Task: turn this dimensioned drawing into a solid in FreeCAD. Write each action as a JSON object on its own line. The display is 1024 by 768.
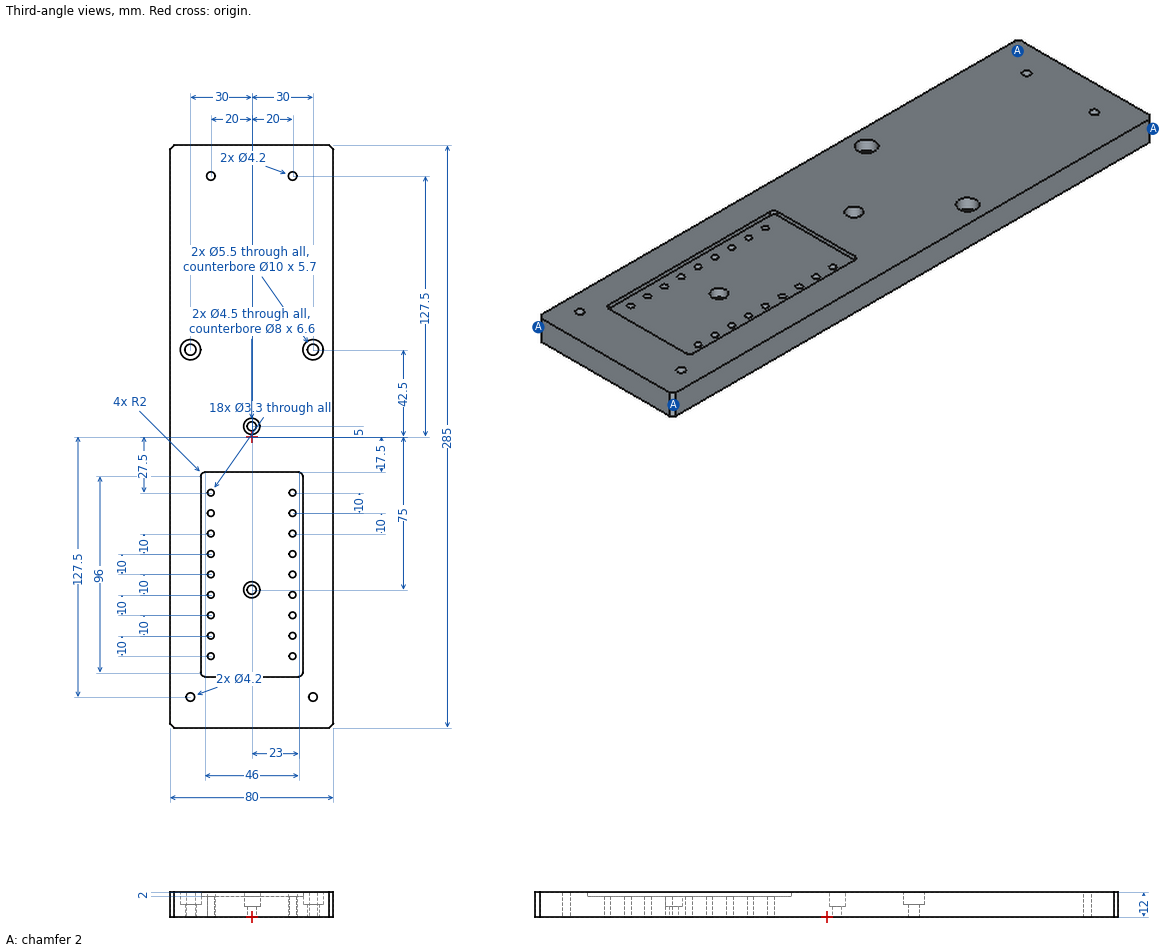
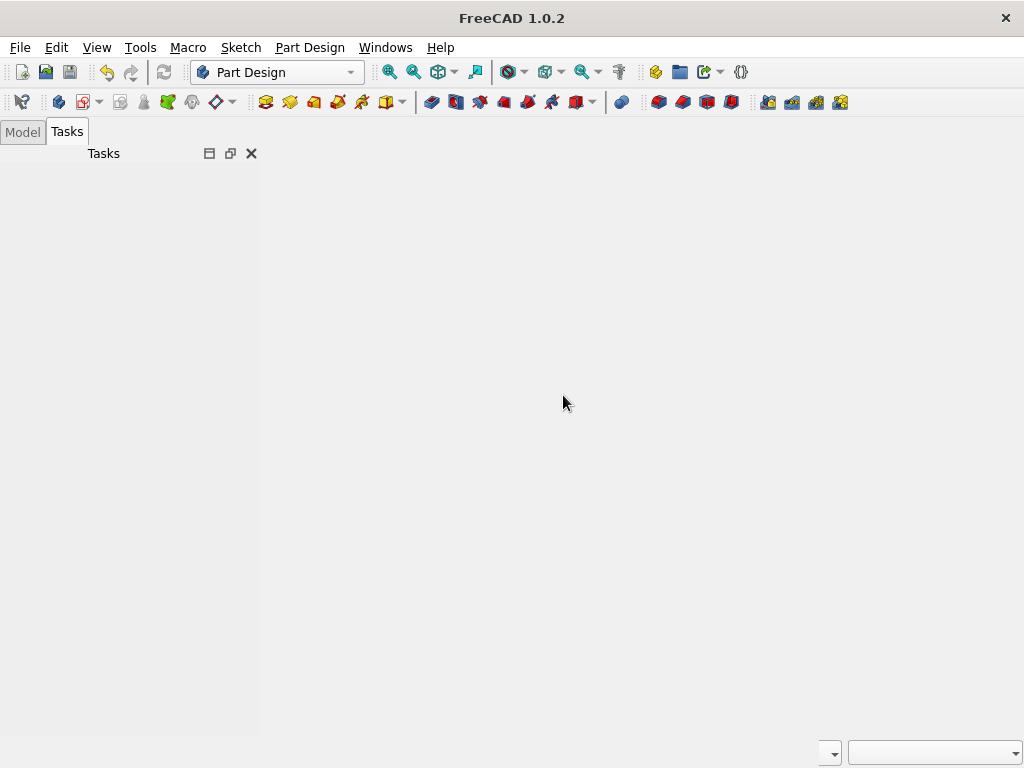
{"action": "key", "text": "ctrl+n"}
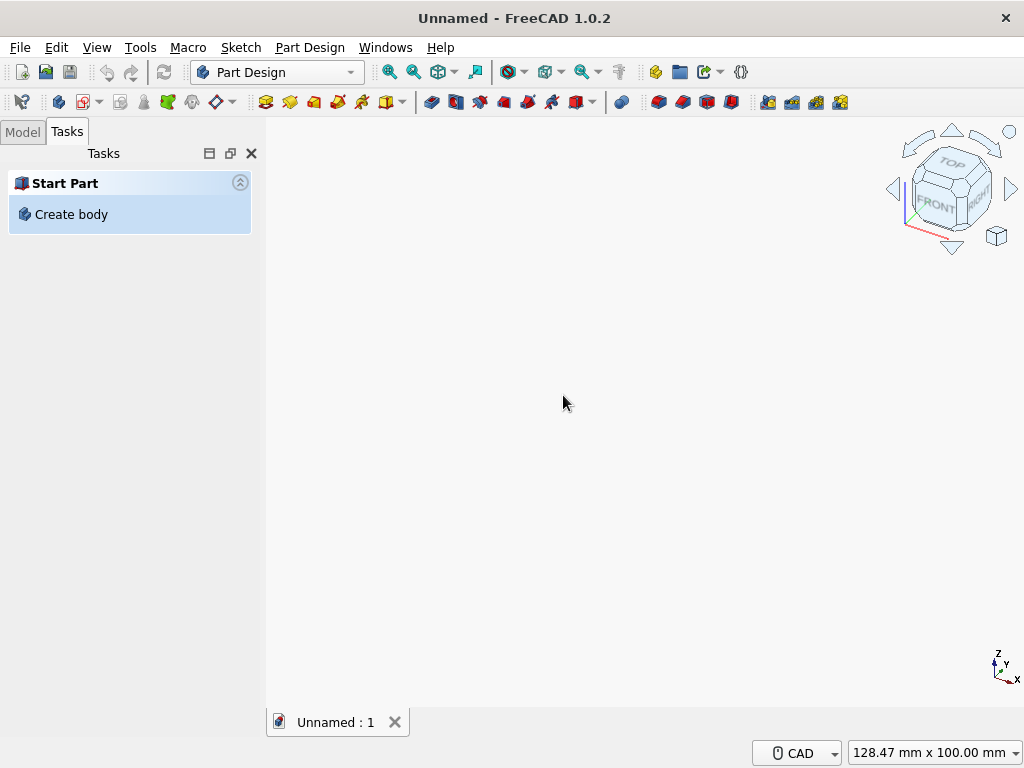
{"action": "left_click", "coordinate": [84, 102]}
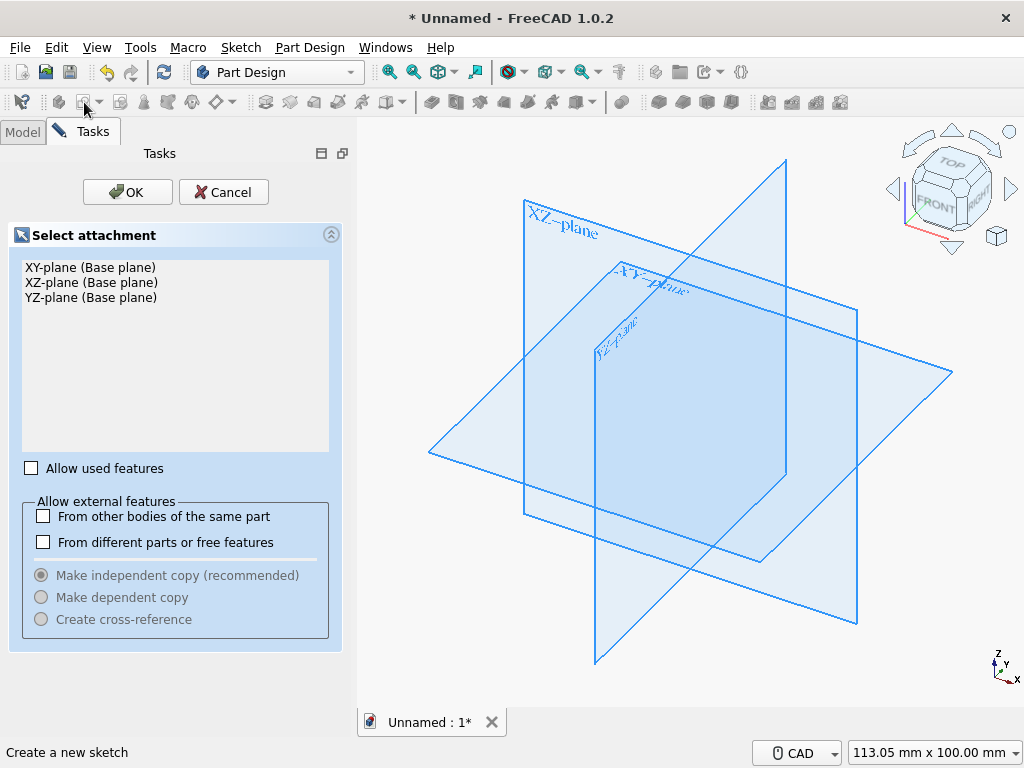
{"action": "left_click", "coordinate": [82, 268]}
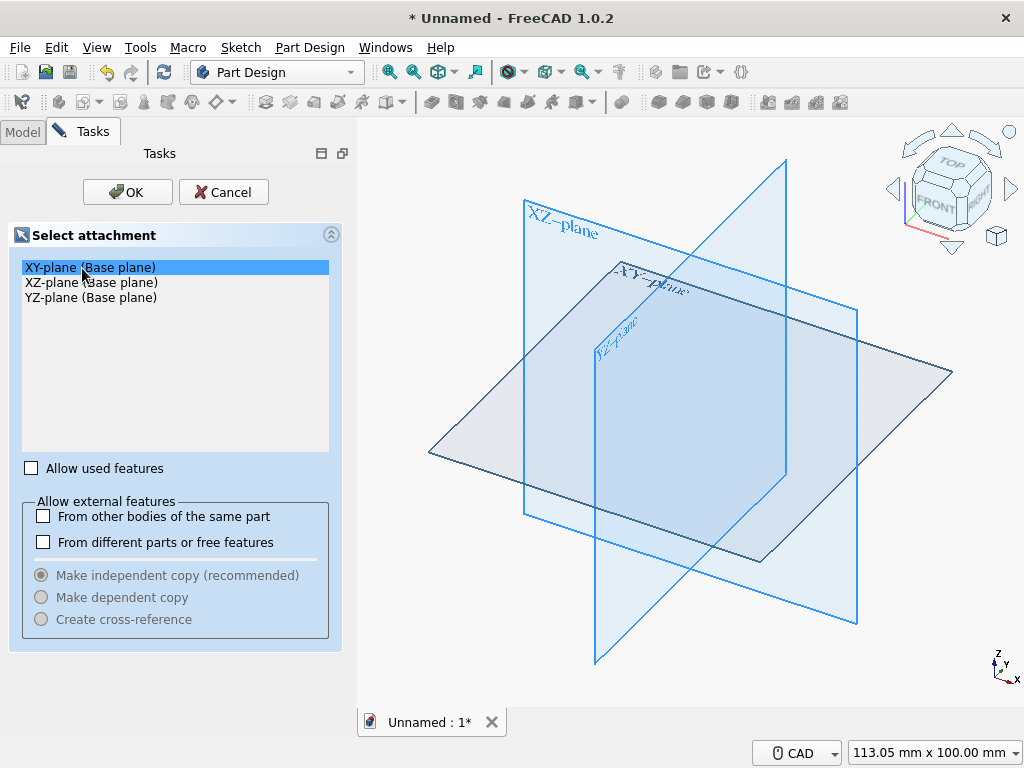
{"action": "left_click", "coordinate": [128, 192]}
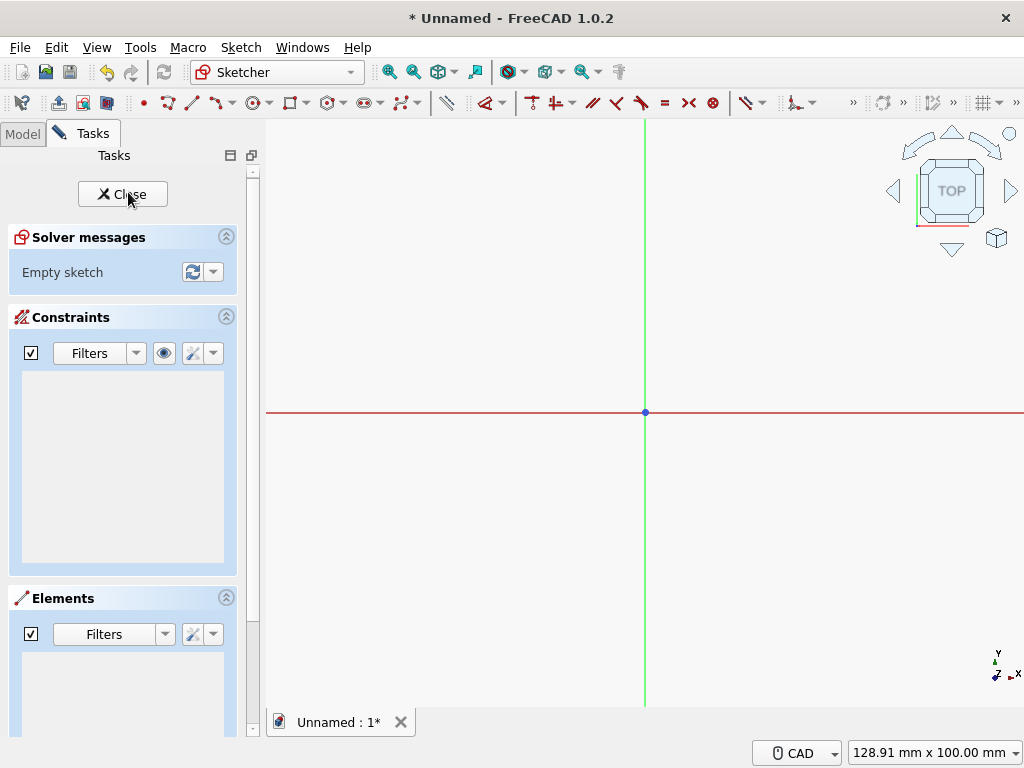
{"action": "scroll", "coordinate": [554, 413], "scroll_direction": "down", "scroll_amount": 7}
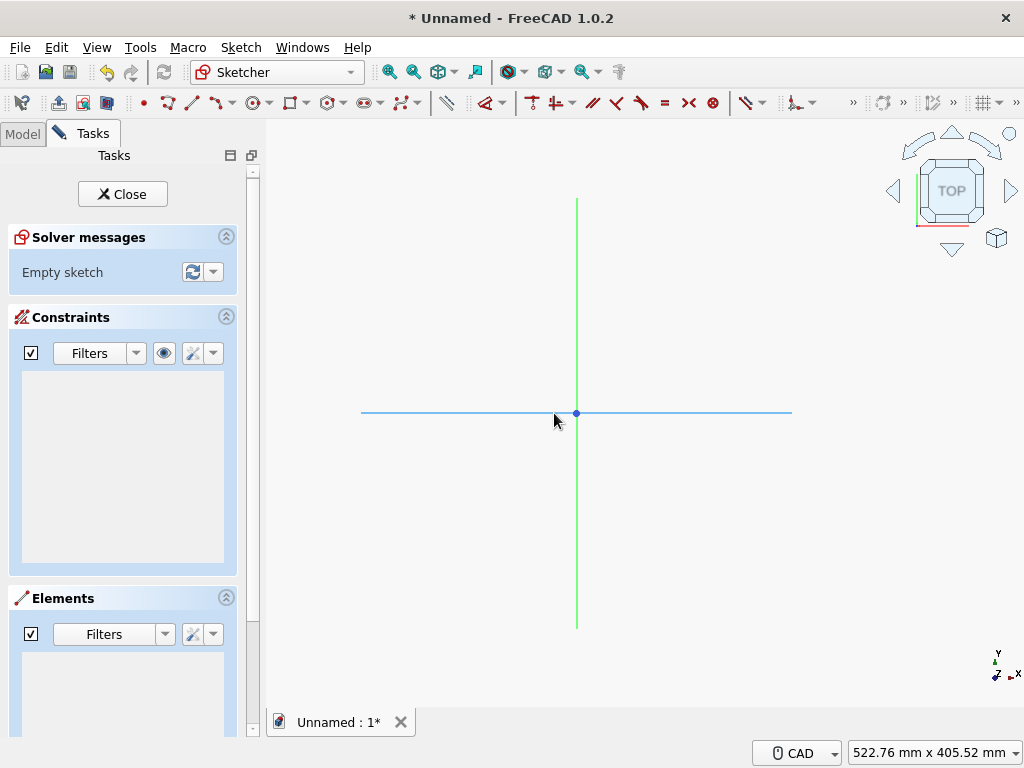
{"action": "key", "text": "g v"}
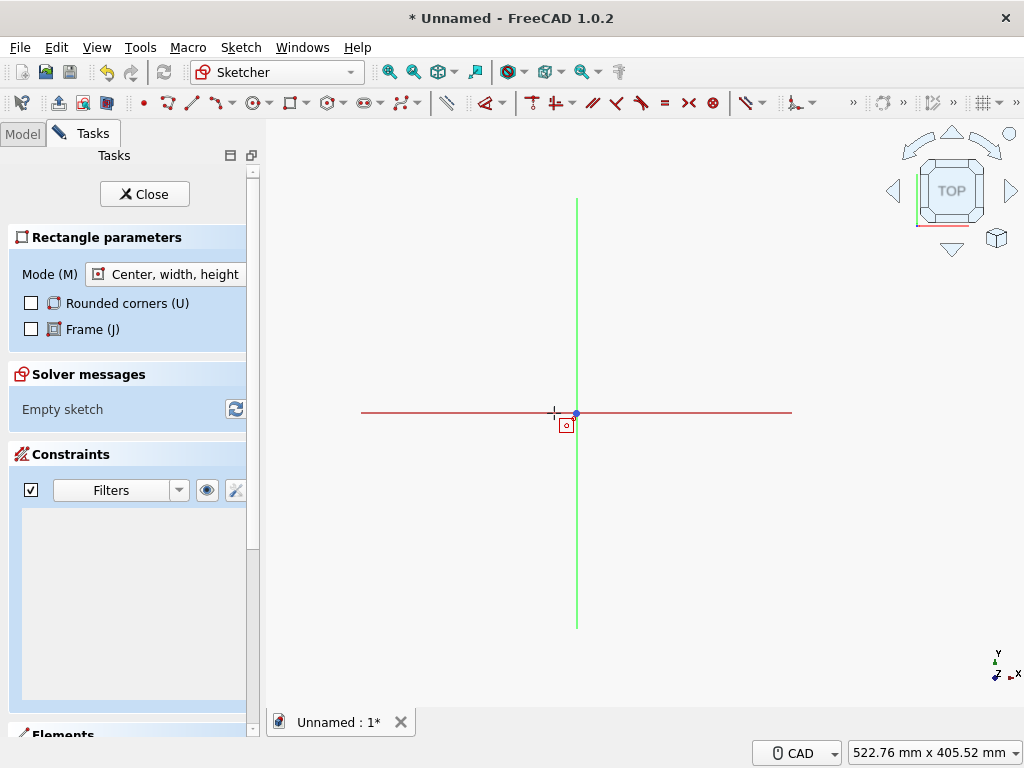
{"action": "left_click", "coordinate": [577, 413]}
{"action": "left_click", "coordinate": [635, 207]}
{"action": "key", "text": "Escape"}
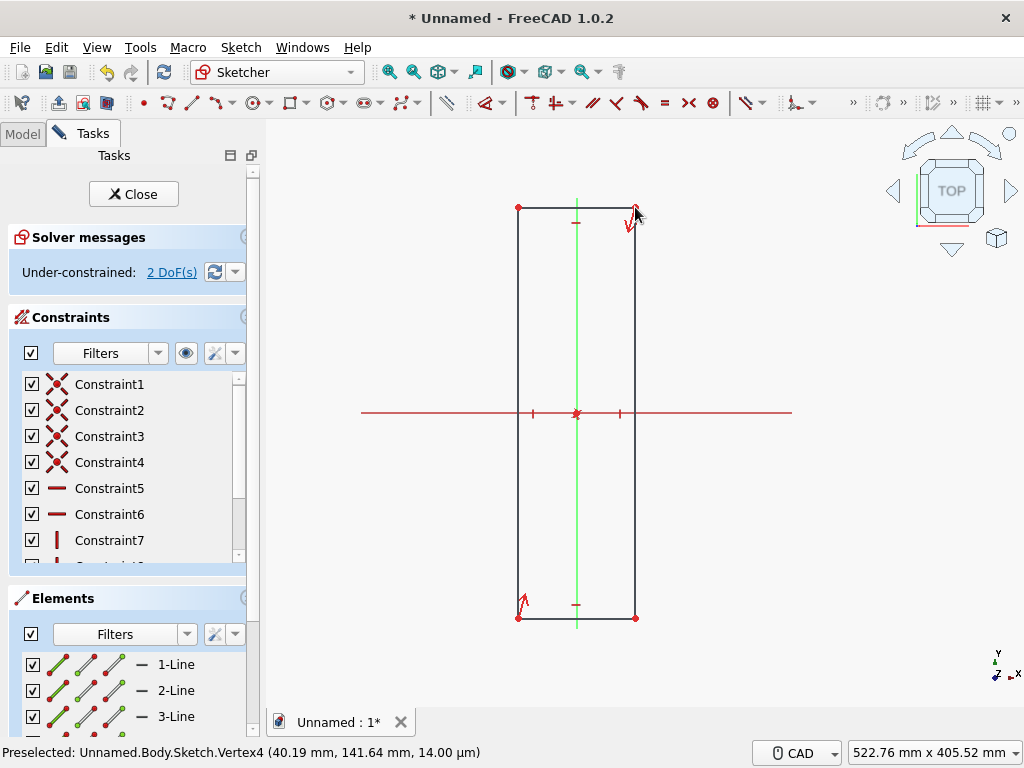
{"action": "key", "text": "d"}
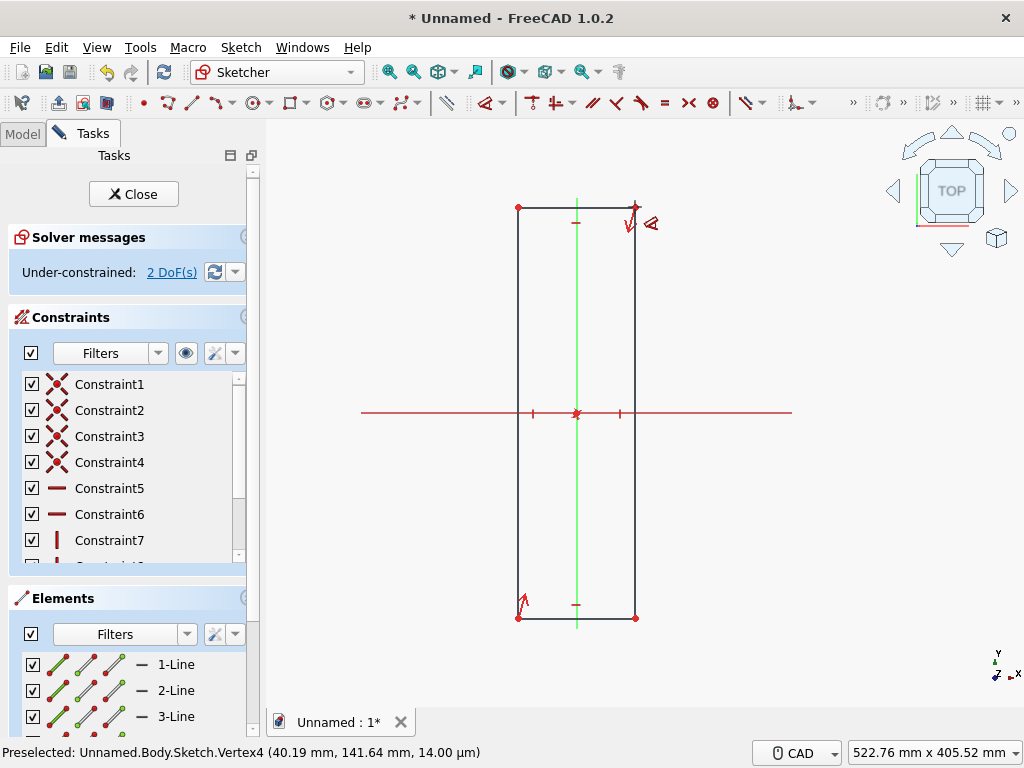
{"action": "left_click", "coordinate": [553, 619]}
{"action": "left_click", "coordinate": [550, 653]}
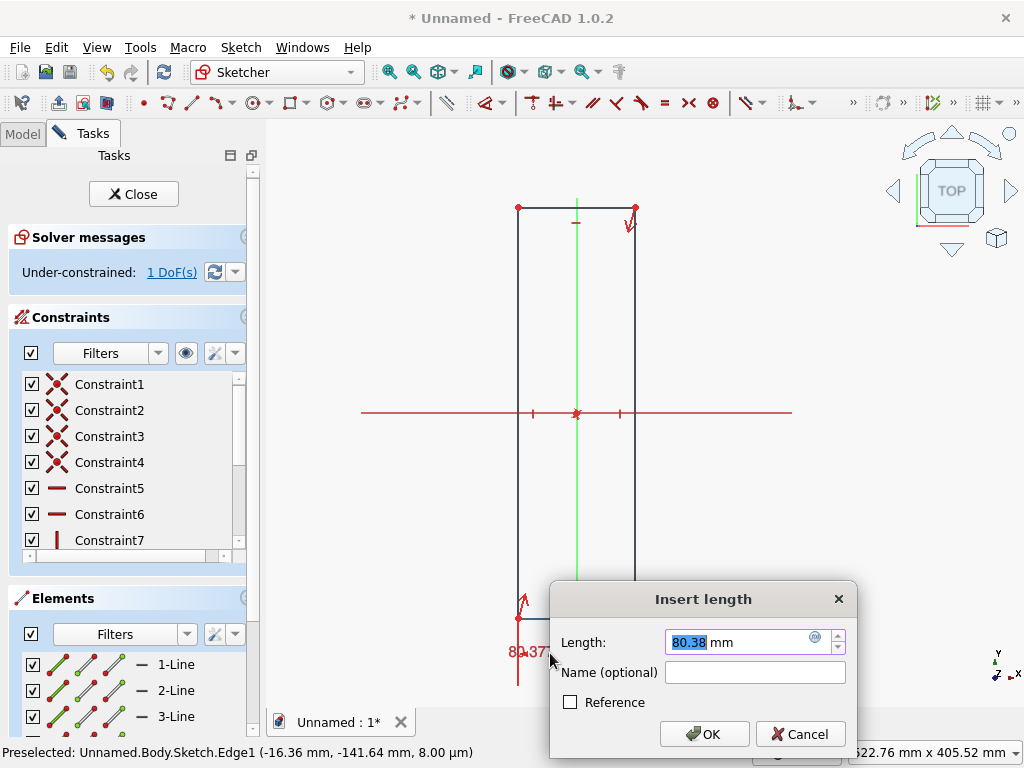
{"action": "type", "text": "80"}
{"action": "key", "text": "Return"}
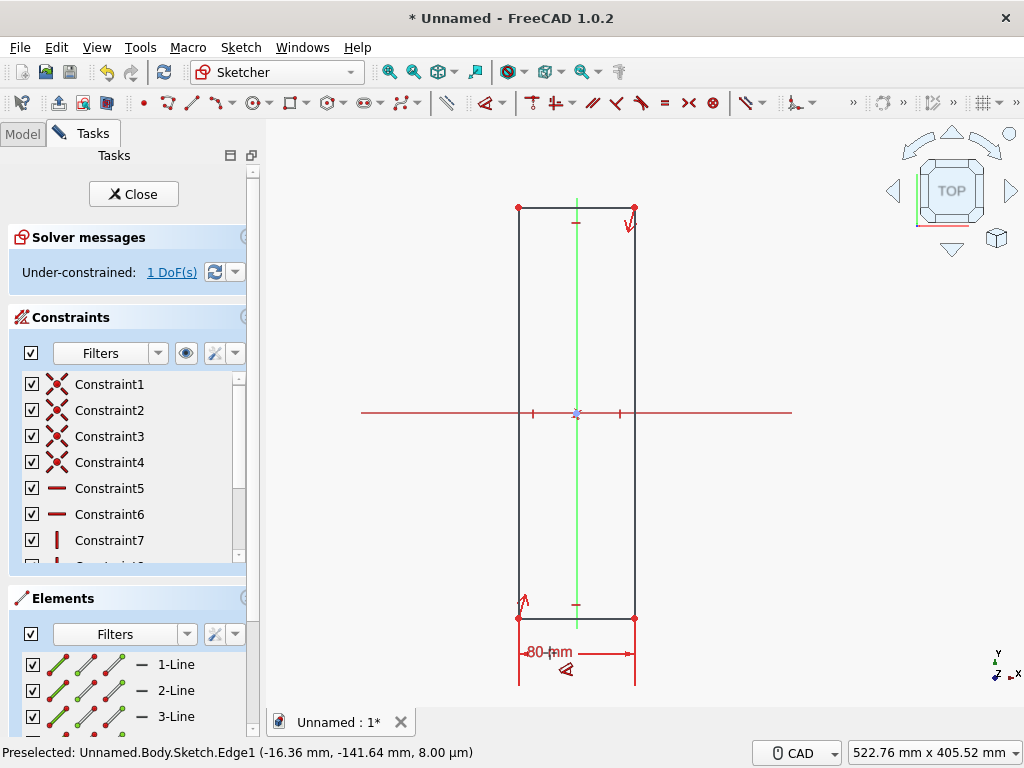
{"action": "left_click", "coordinate": [635, 496]}
{"action": "left_click", "coordinate": [669, 319]}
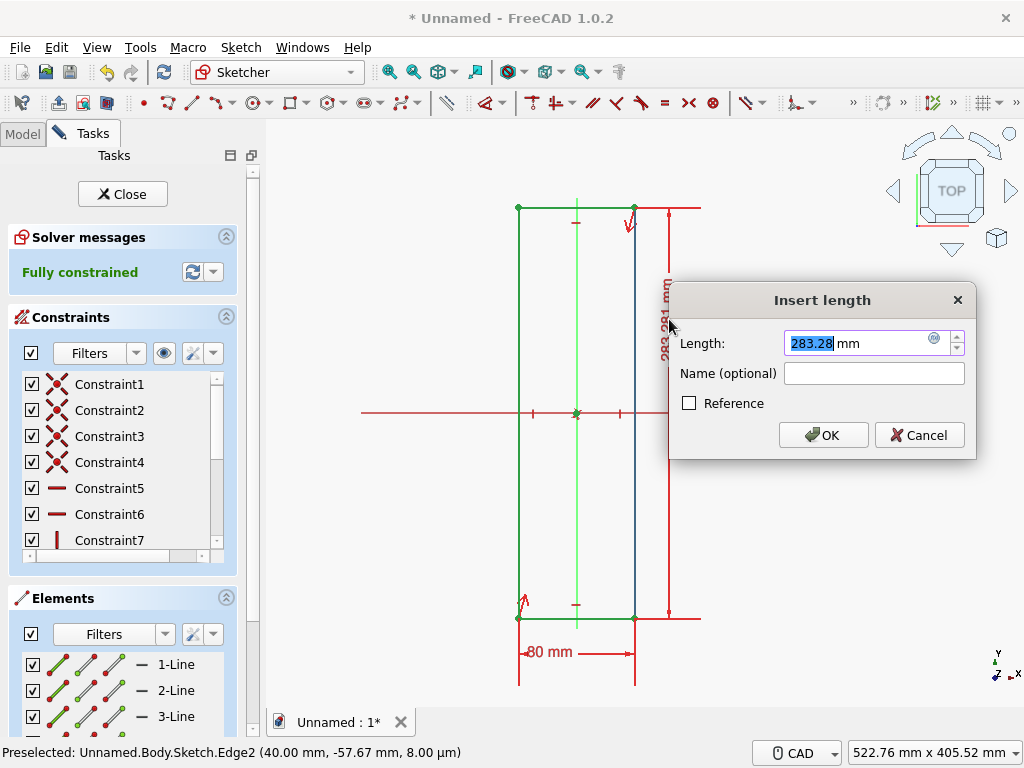
{"action": "type", "text": "285"}
{"action": "key", "text": "Return"}
{"action": "key", "text": "Escape"}